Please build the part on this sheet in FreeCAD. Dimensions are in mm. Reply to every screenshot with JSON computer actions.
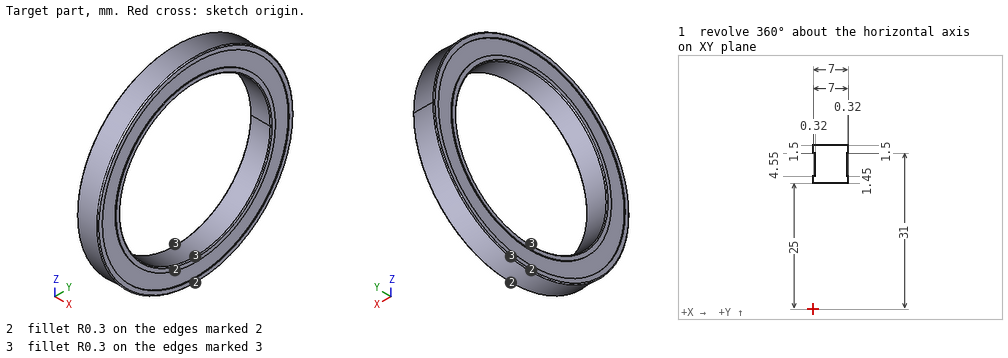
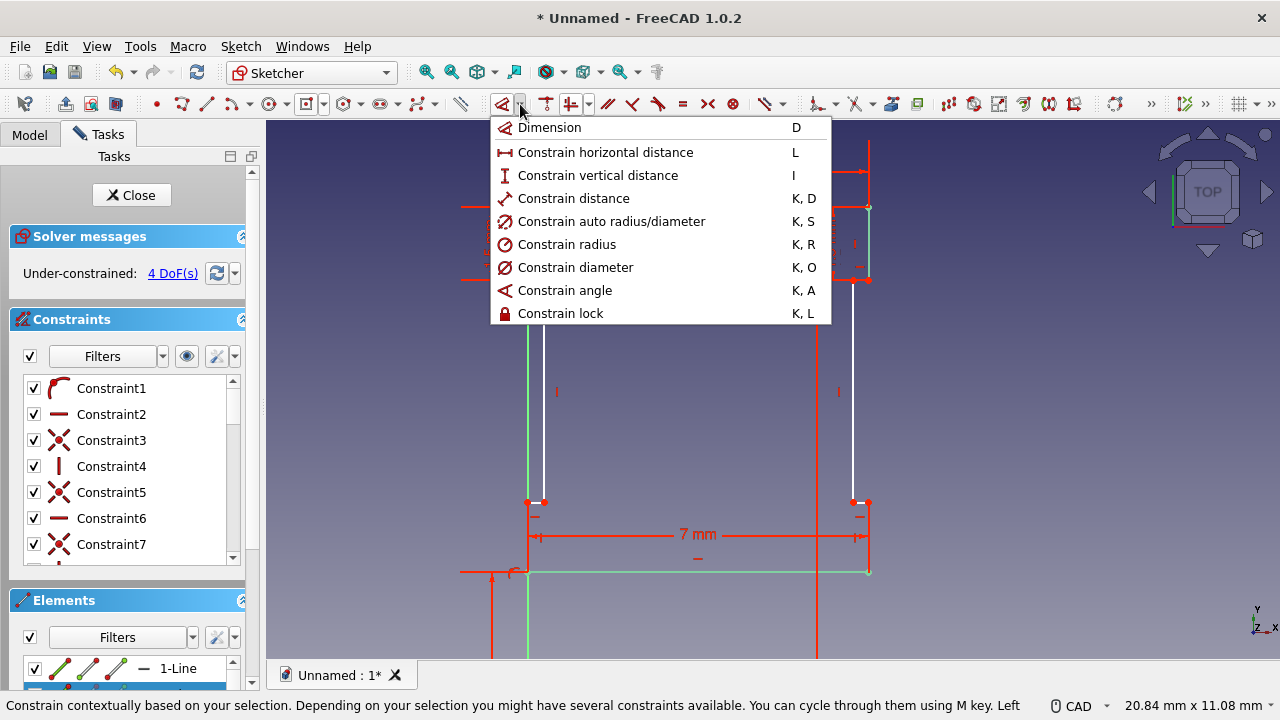
{"action": "left_click", "coordinate": [661, 176]}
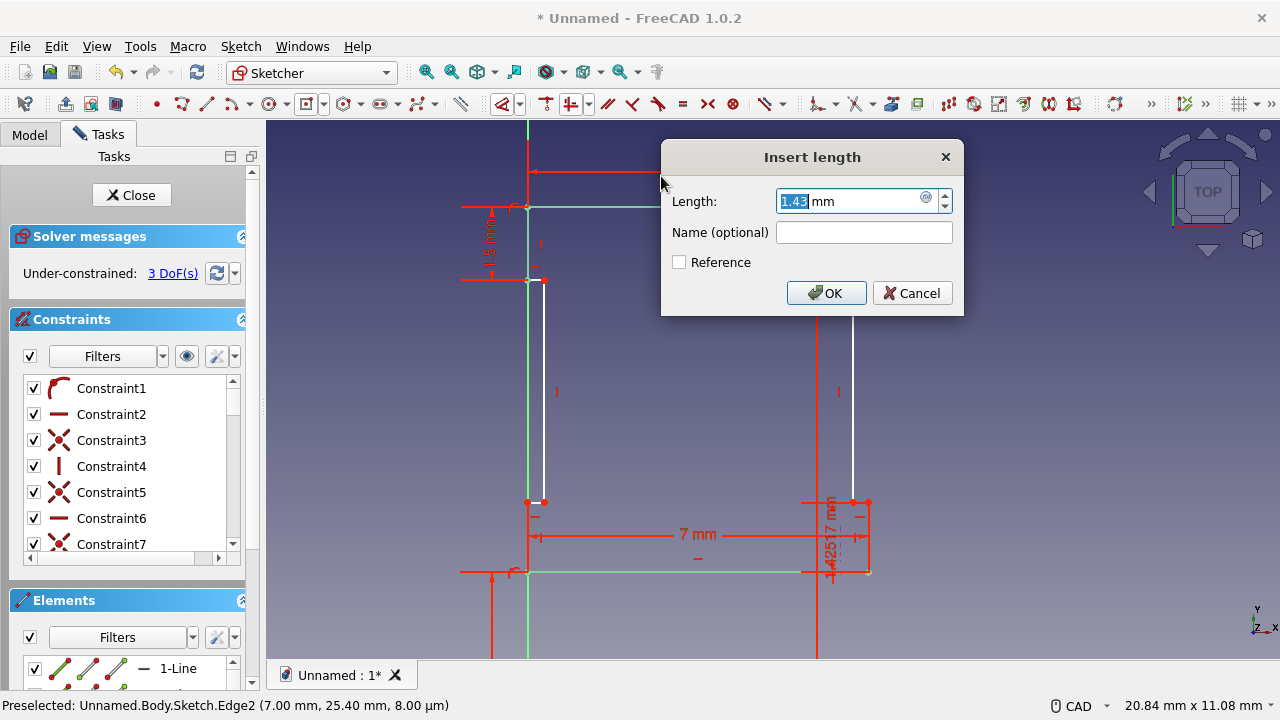
{"action": "type", "text": "1.45"}
{"action": "key", "text": "Return"}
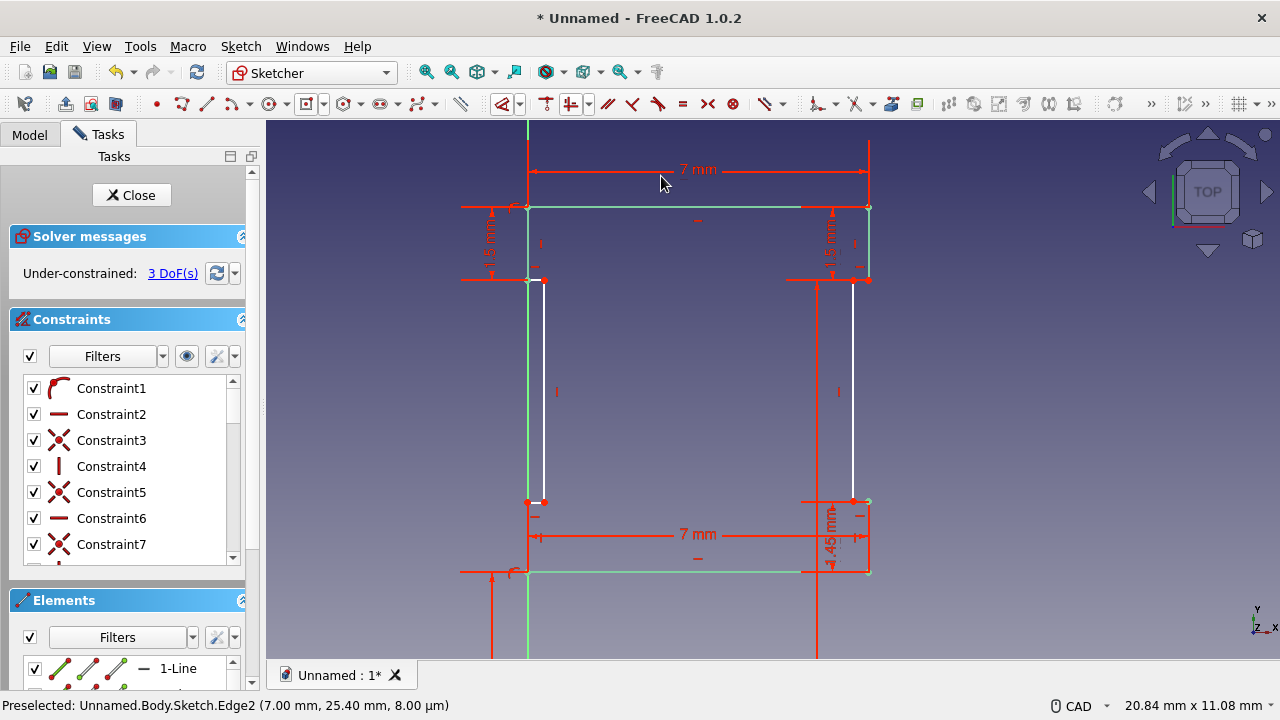
{"action": "scroll", "coordinate": [861, 502], "scroll_direction": "up", "scroll_amount": 5}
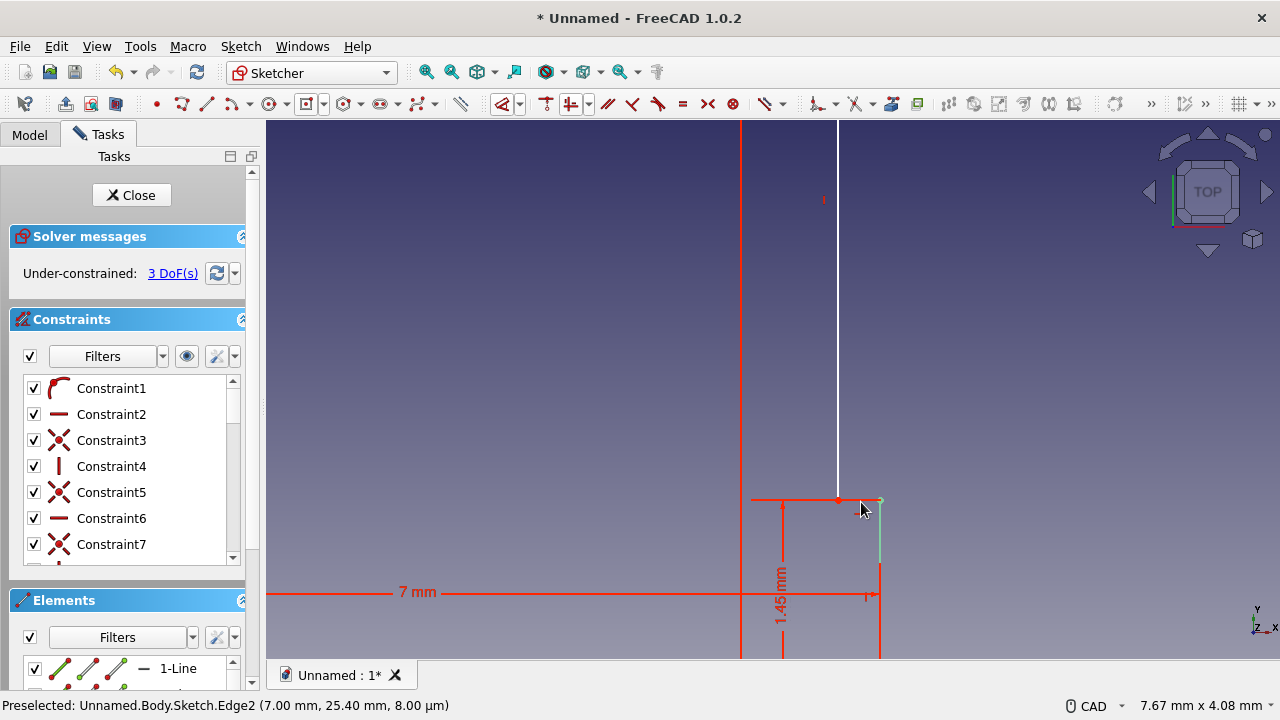
{"action": "left_click", "coordinate": [859, 500]}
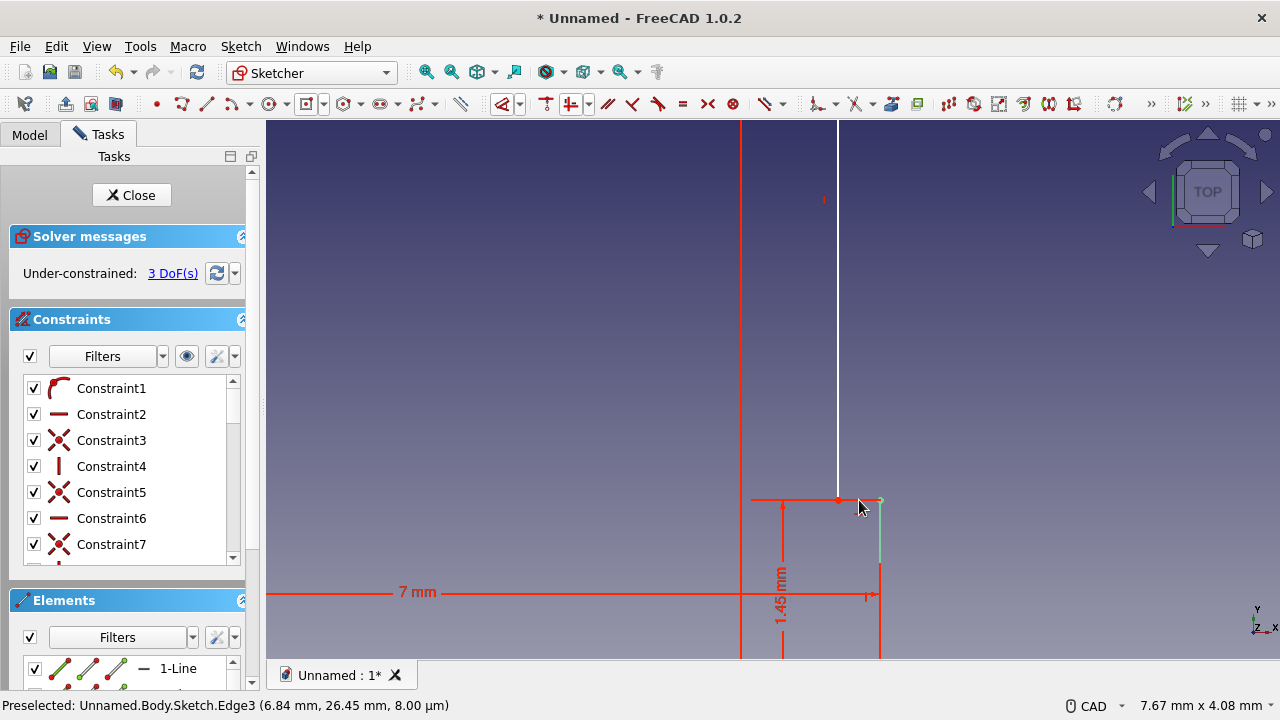
{"action": "key", "text": "l"}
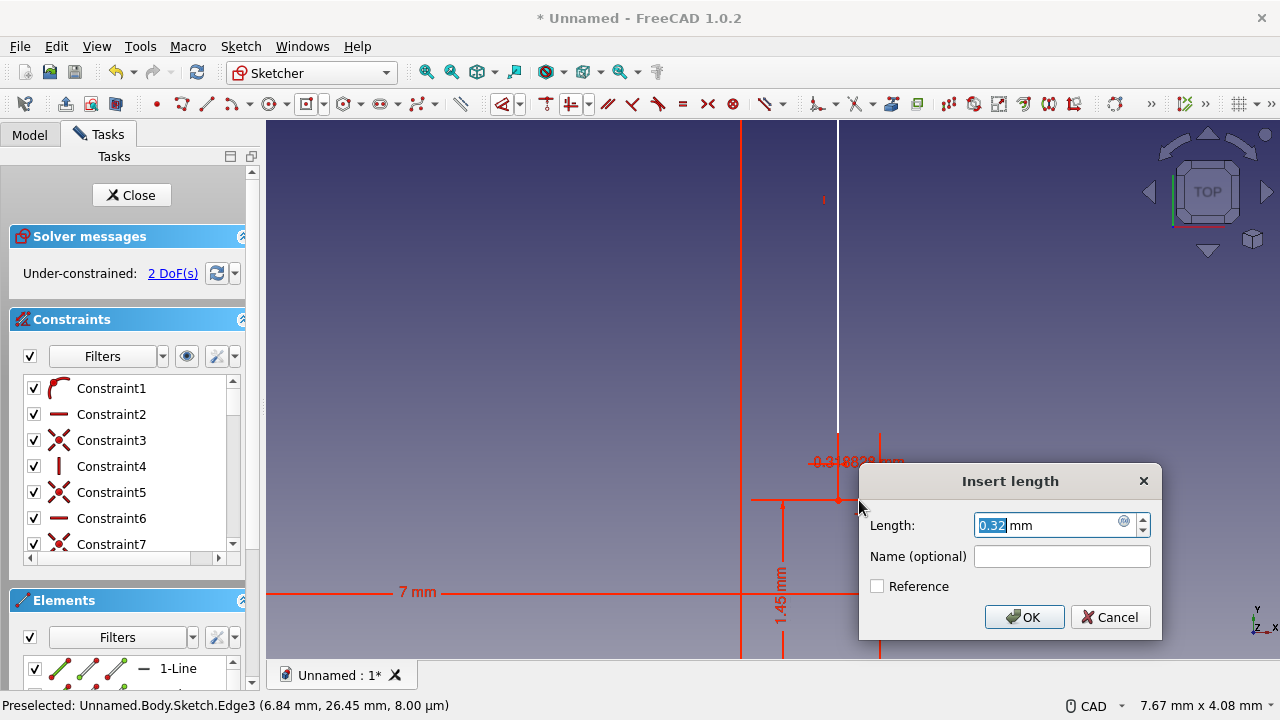
{"action": "type", "text": "0.32"}
{"action": "key", "text": "Return"}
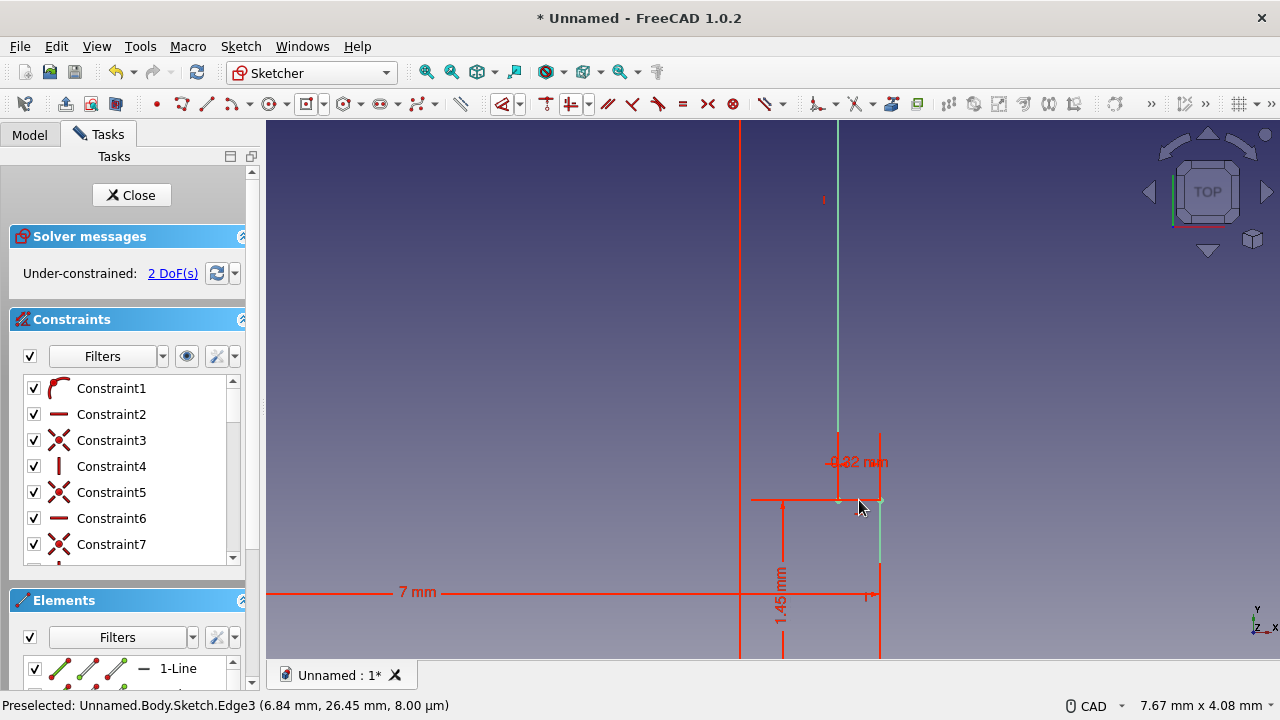
{"action": "scroll", "coordinate": [871, 502], "scroll_direction": "down", "scroll_amount": 5}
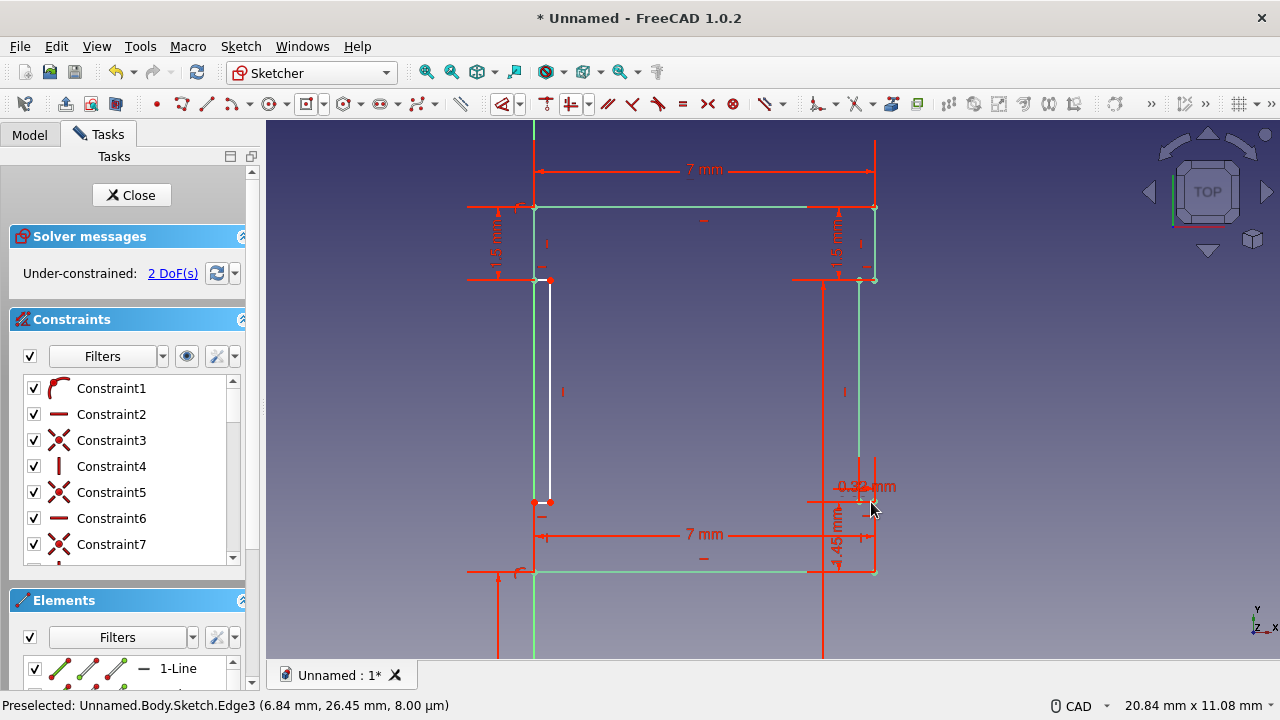
{"action": "scroll", "coordinate": [539, 280], "scroll_direction": "up", "scroll_amount": 6}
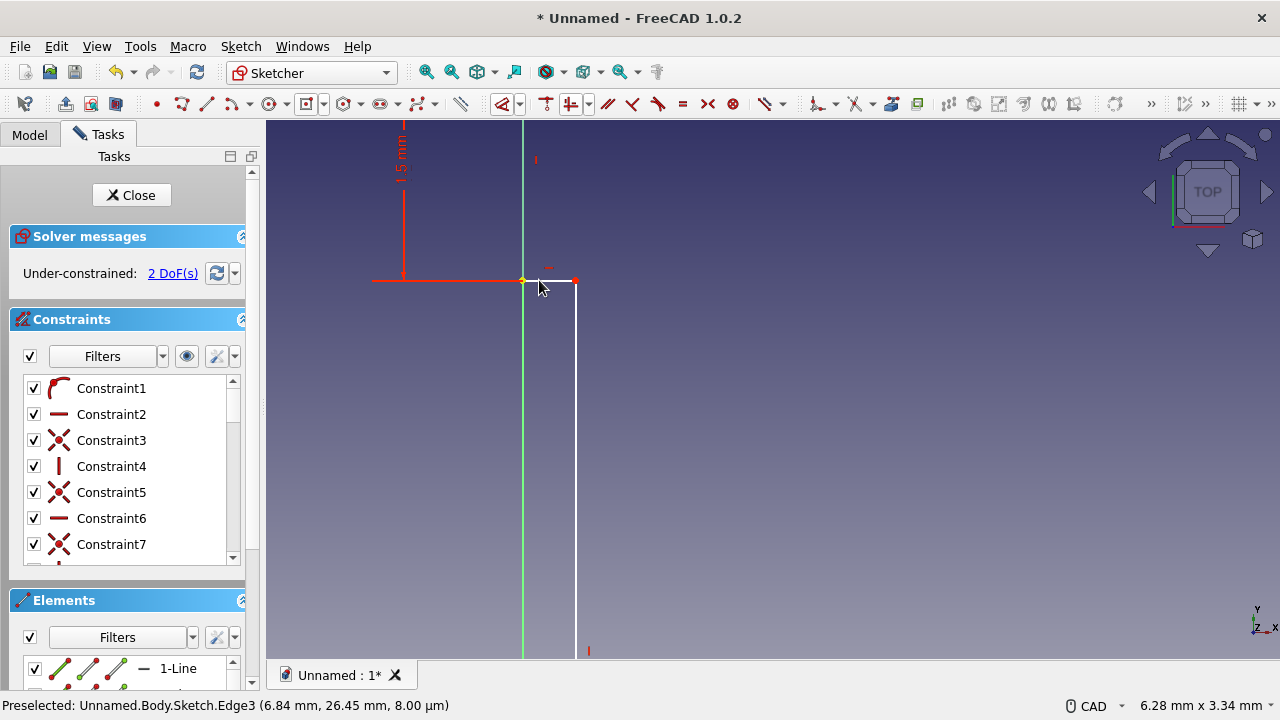
{"action": "left_click", "coordinate": [539, 281]}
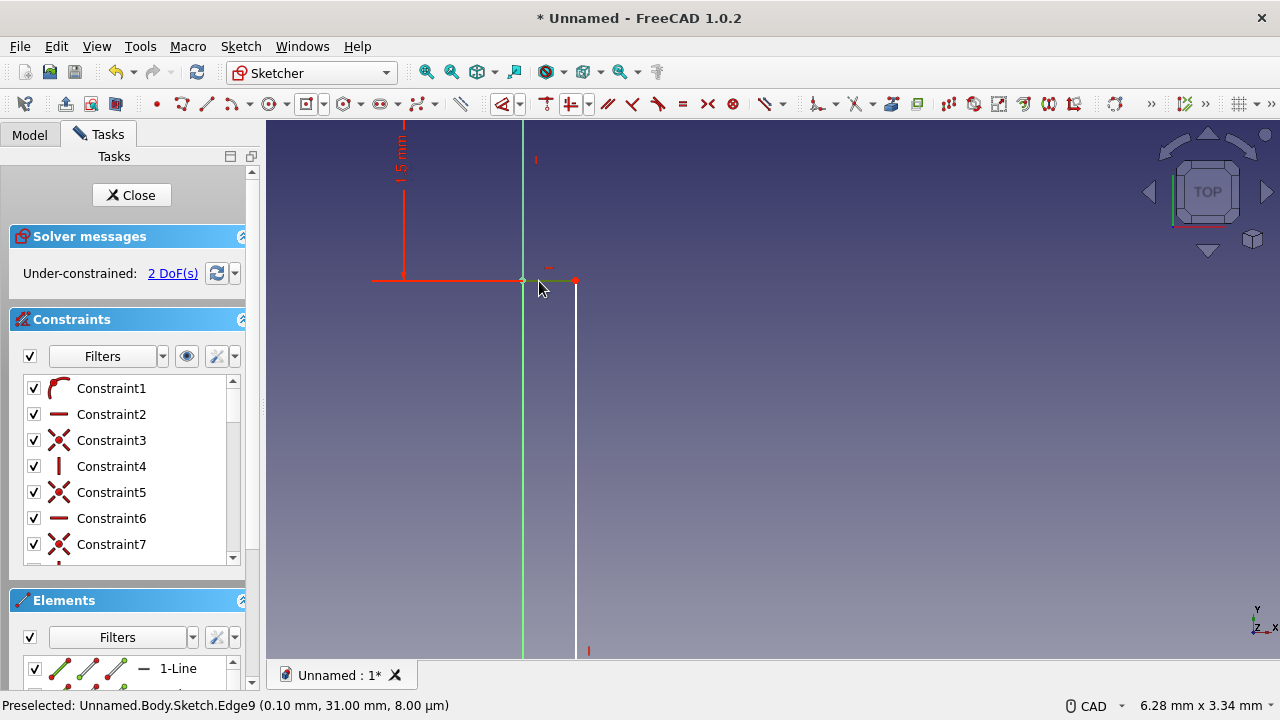
{"action": "left_click", "coordinate": [520, 104]}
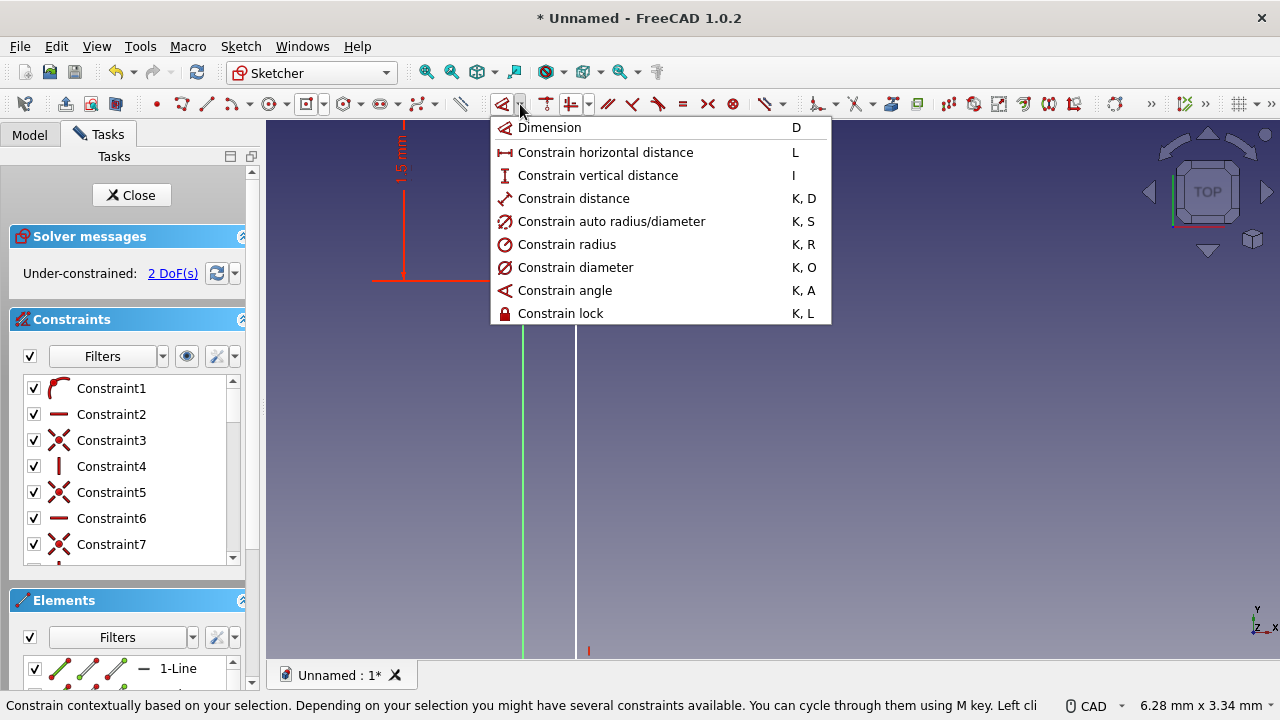
{"action": "left_click", "coordinate": [661, 152]}